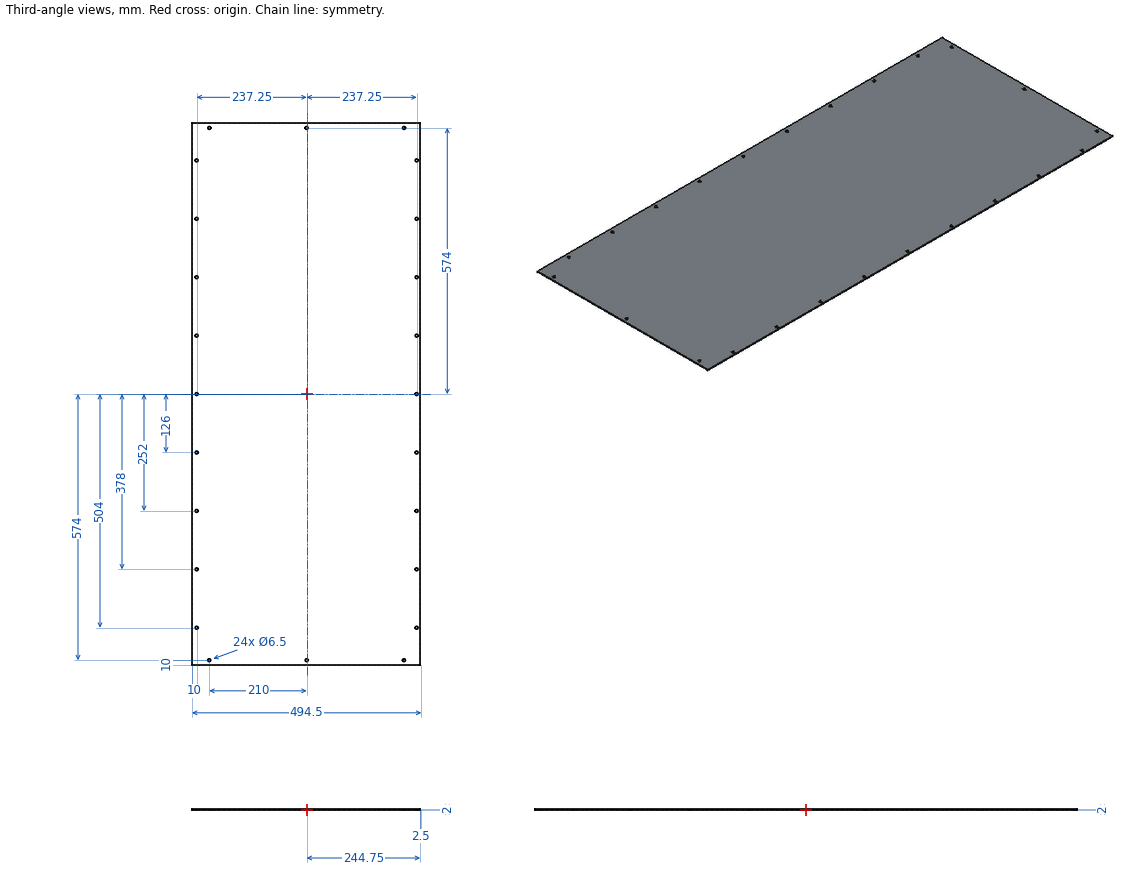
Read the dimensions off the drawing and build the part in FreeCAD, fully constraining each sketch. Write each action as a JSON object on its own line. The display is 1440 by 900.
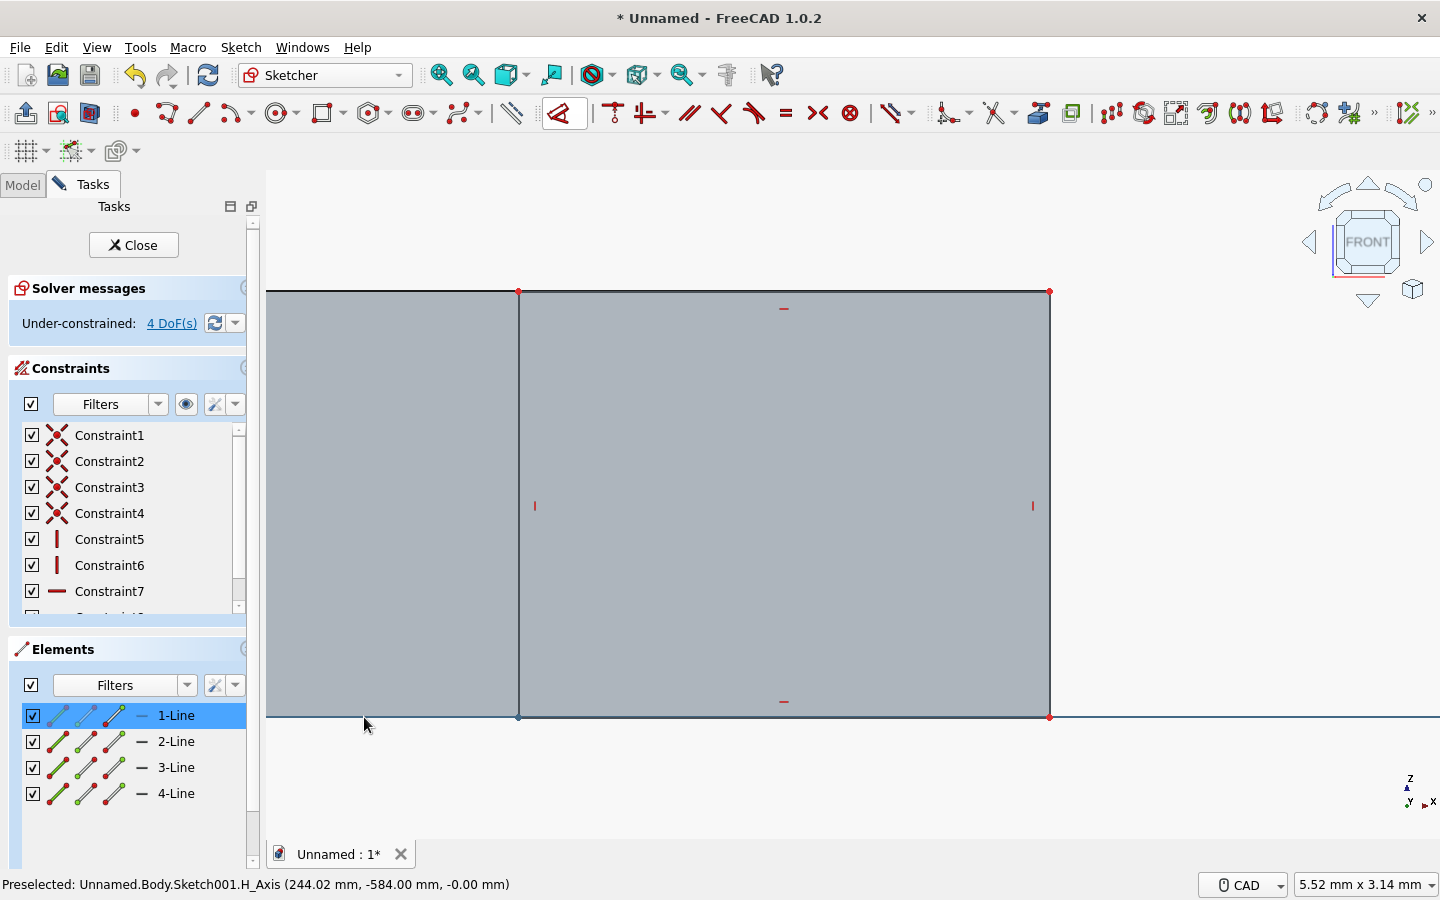
{"action": "left_click", "coordinate": [614, 114]}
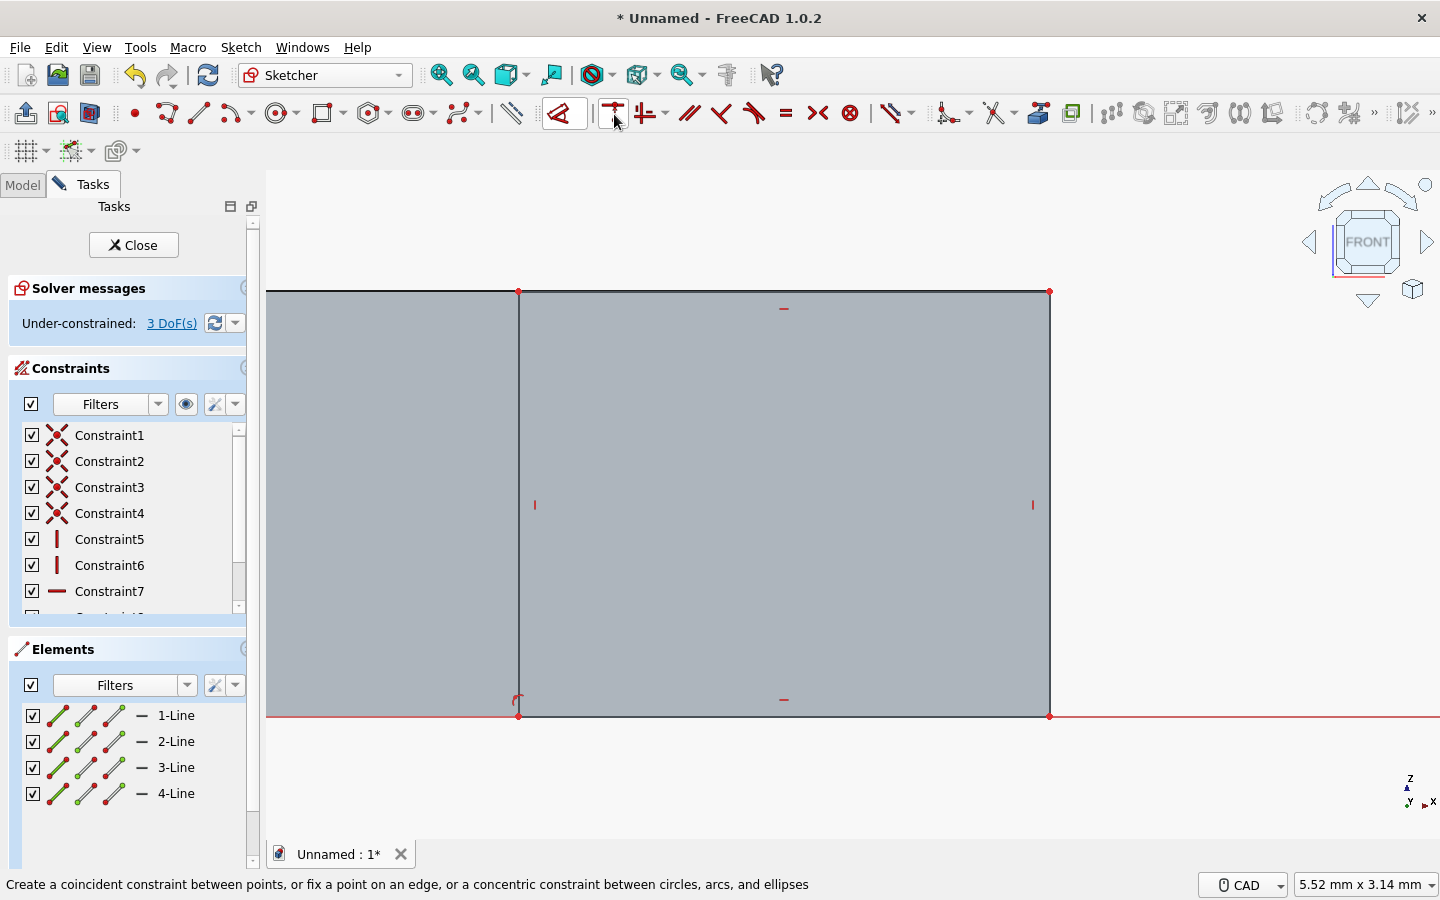
{"action": "left_click", "coordinate": [519, 419]}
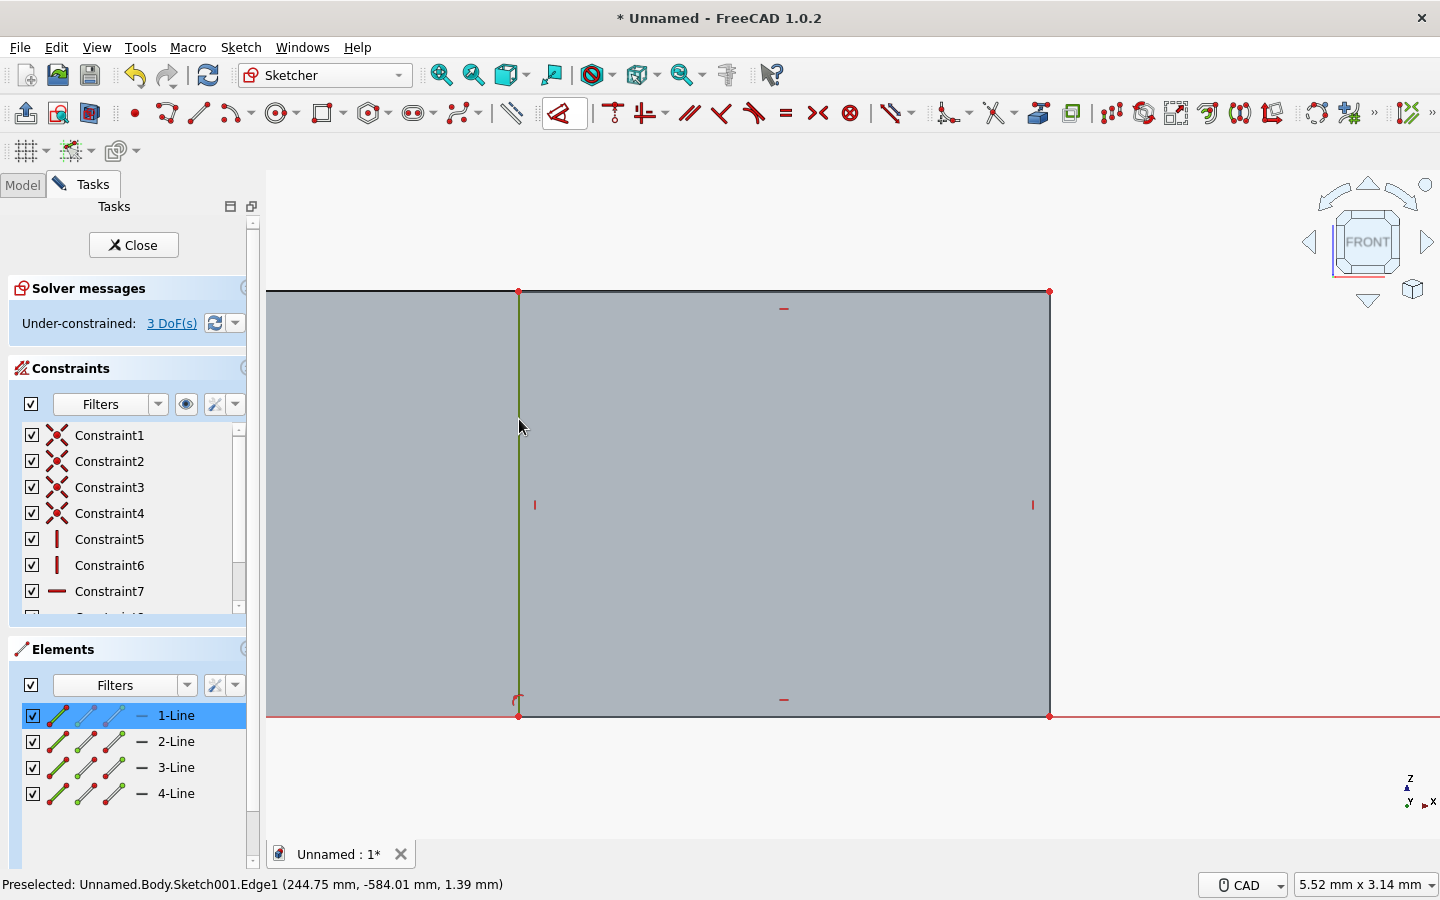
{"action": "key", "text": "i"}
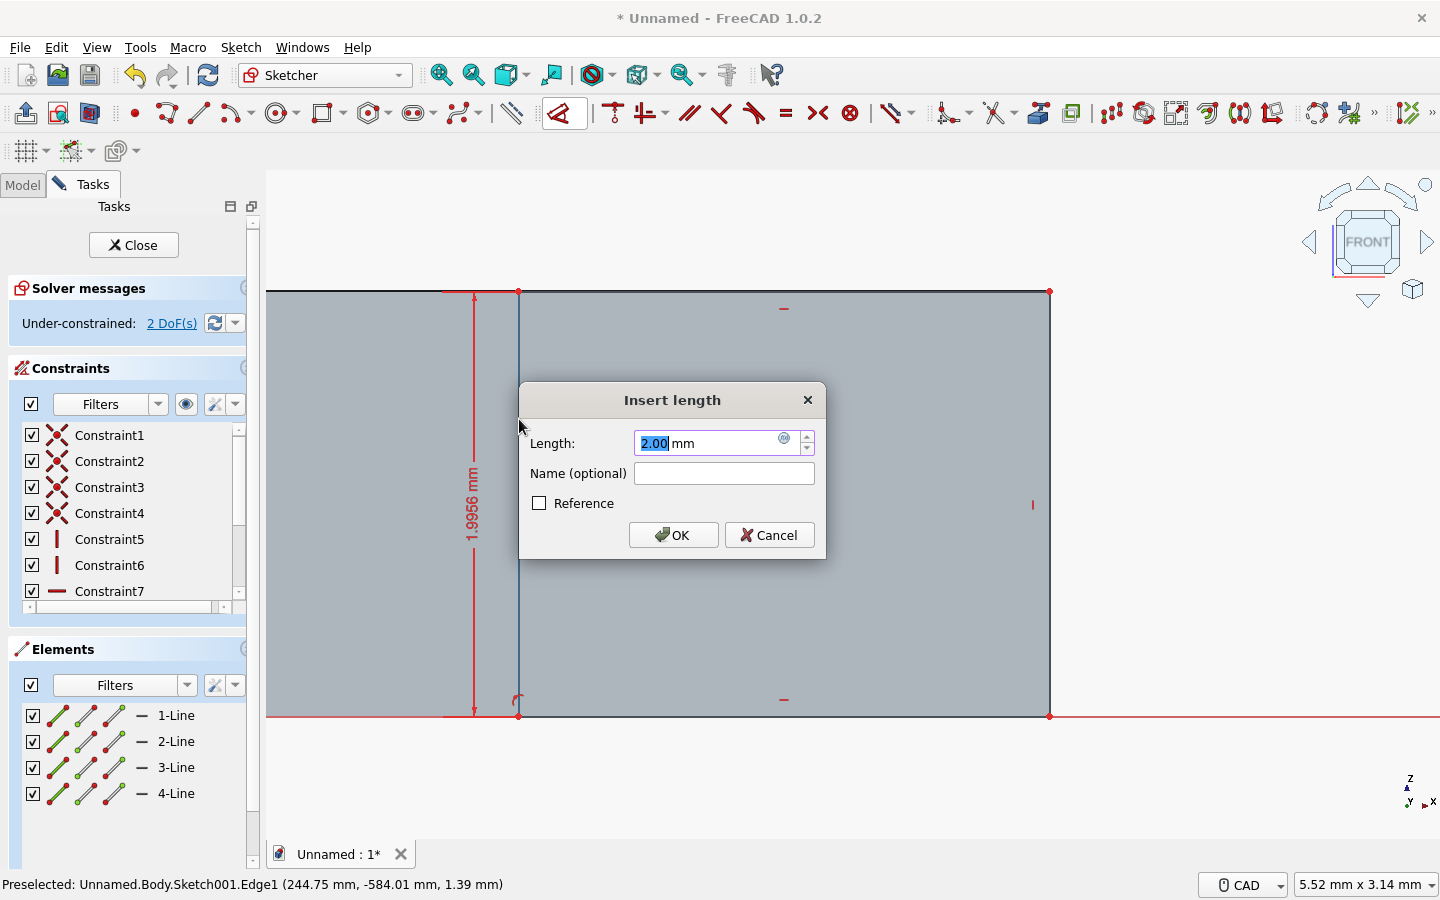
{"action": "type", "text": "2"}
{"action": "key", "text": "Return"}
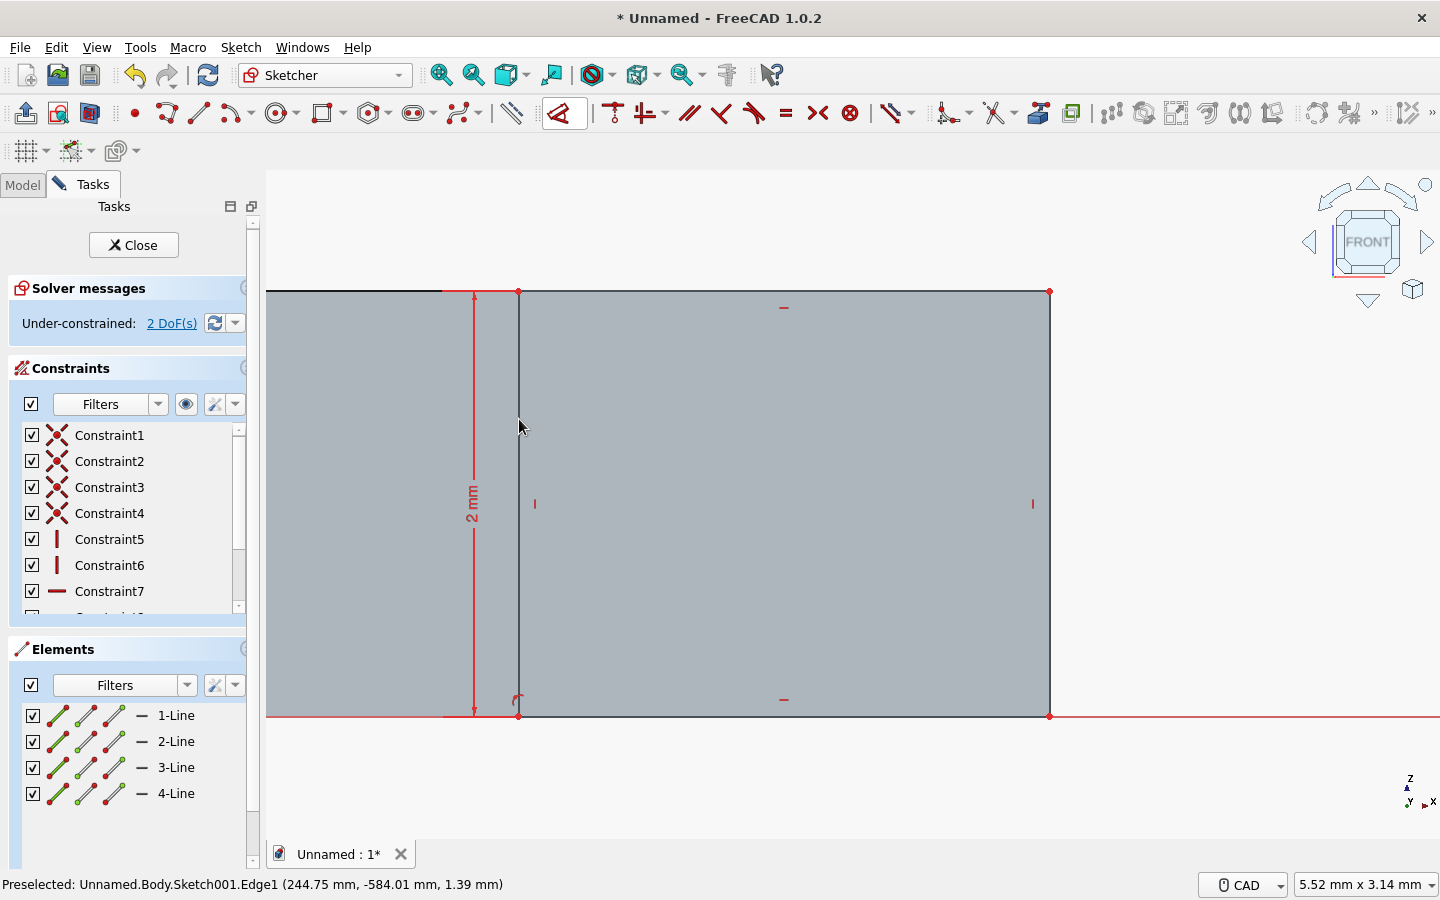
{"action": "left_click", "coordinate": [678, 717]}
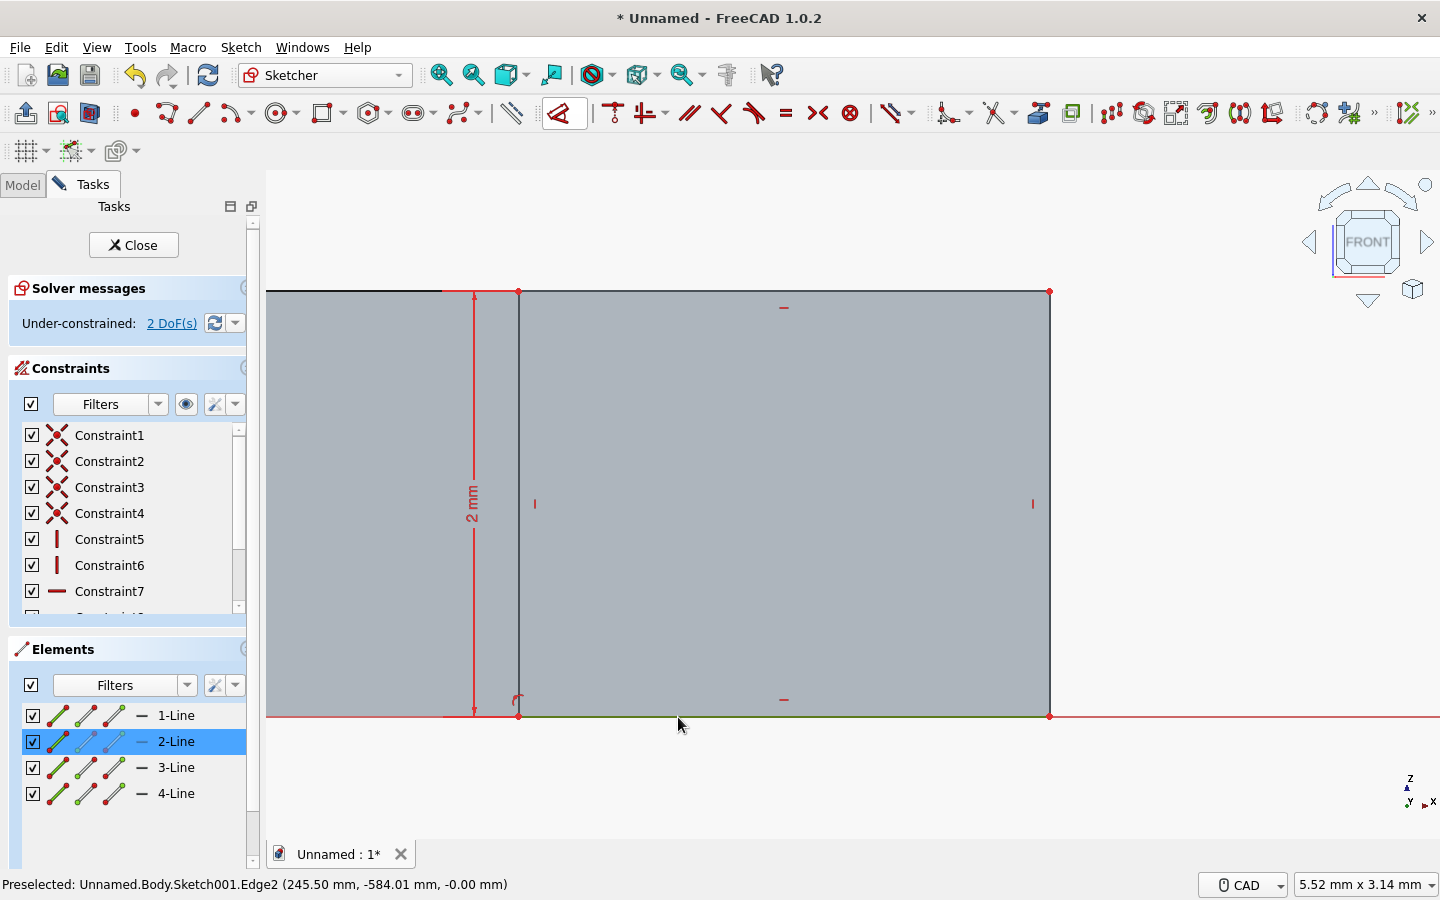
{"action": "key", "text": "l"}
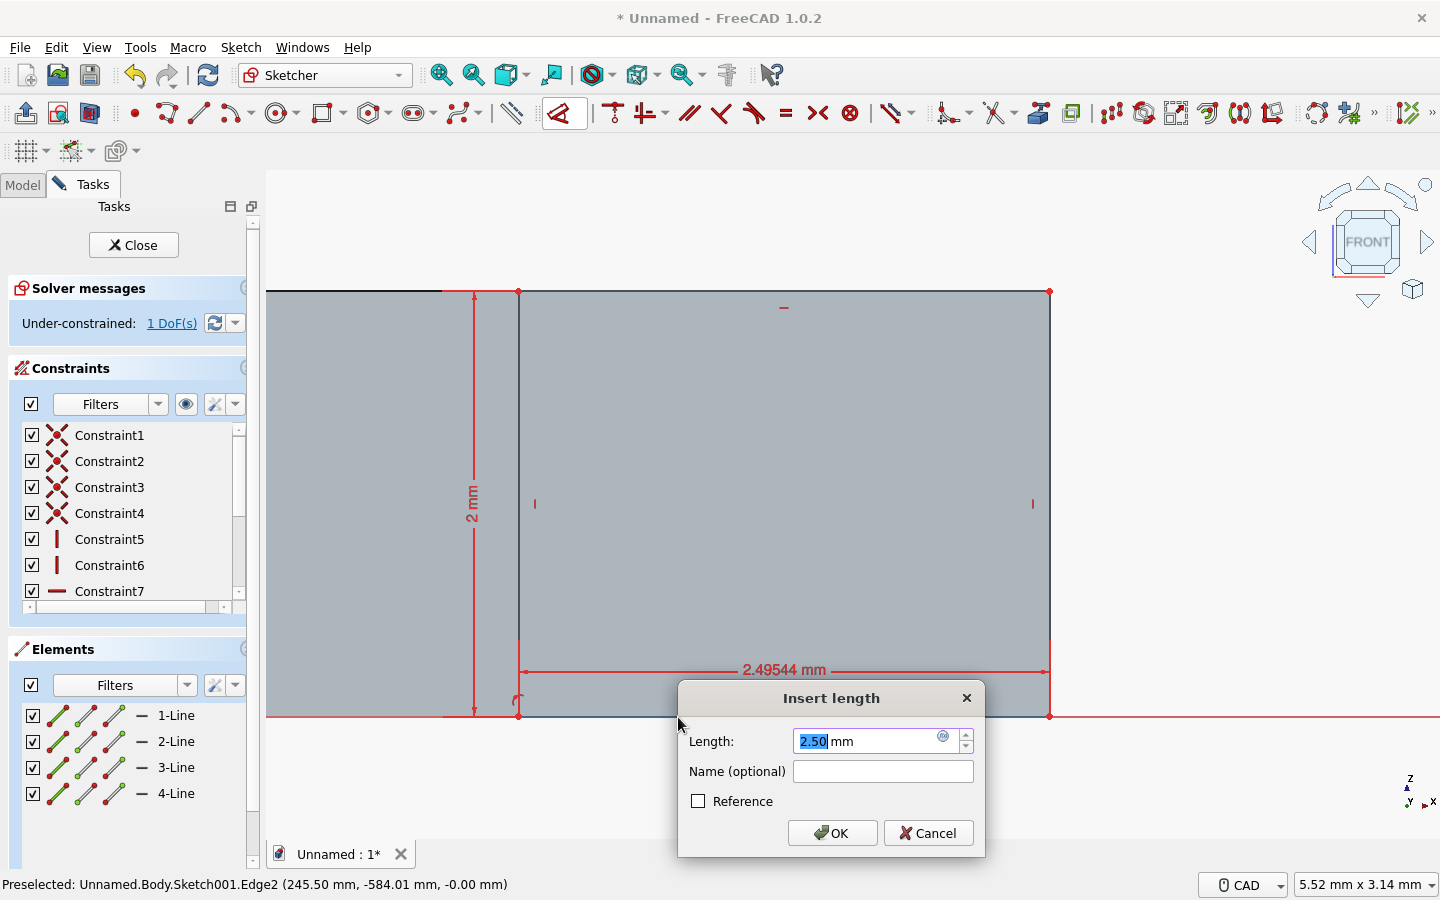
{"action": "type", "text": "2.5"}
{"action": "key", "text": "Return"}